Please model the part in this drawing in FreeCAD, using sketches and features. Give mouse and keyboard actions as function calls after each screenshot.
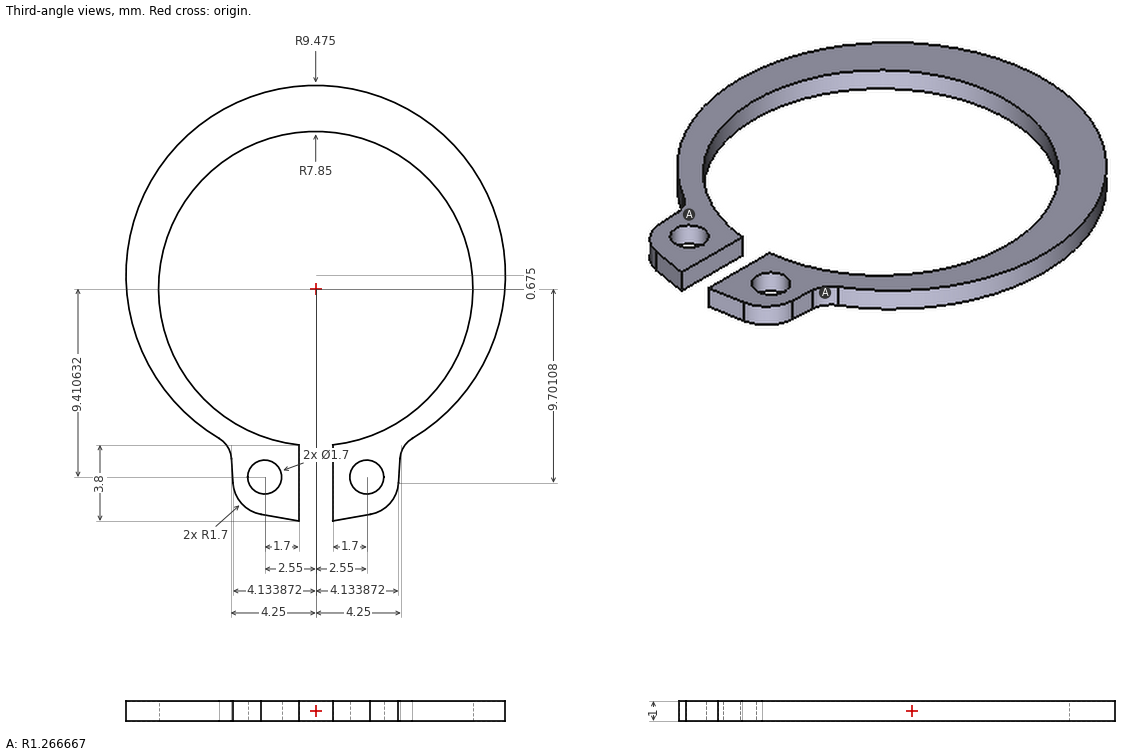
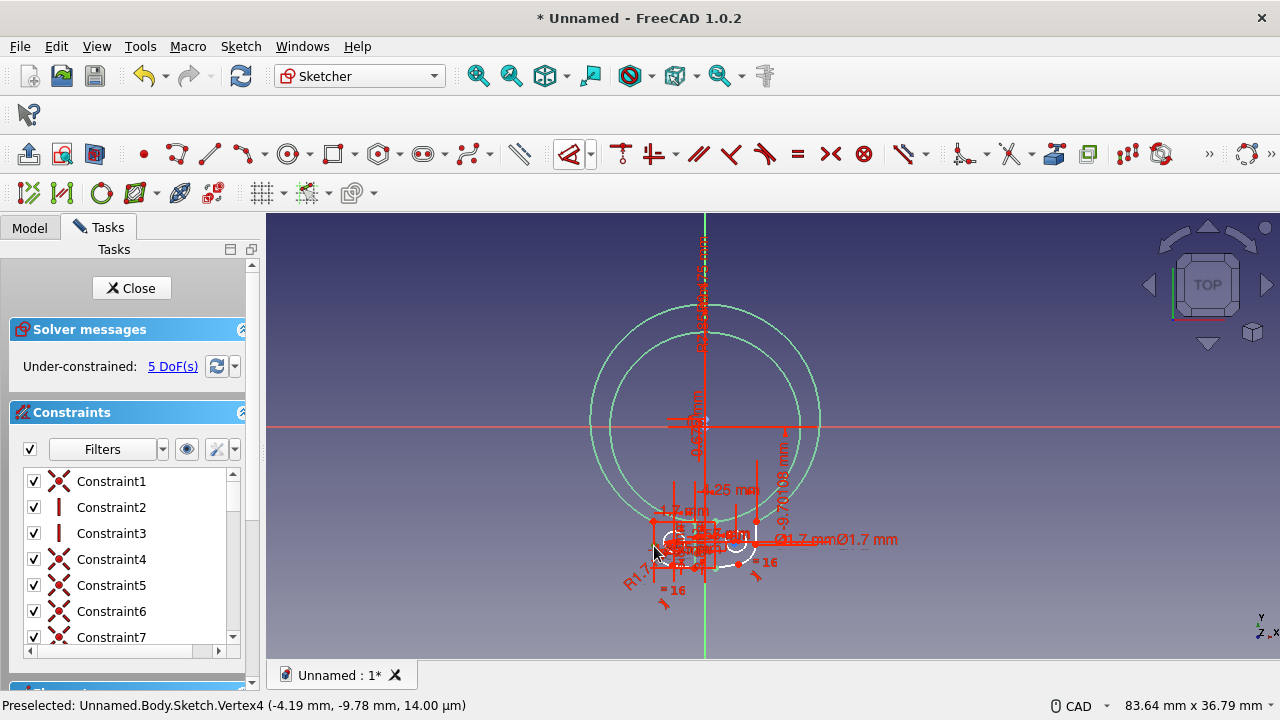
click(590, 154)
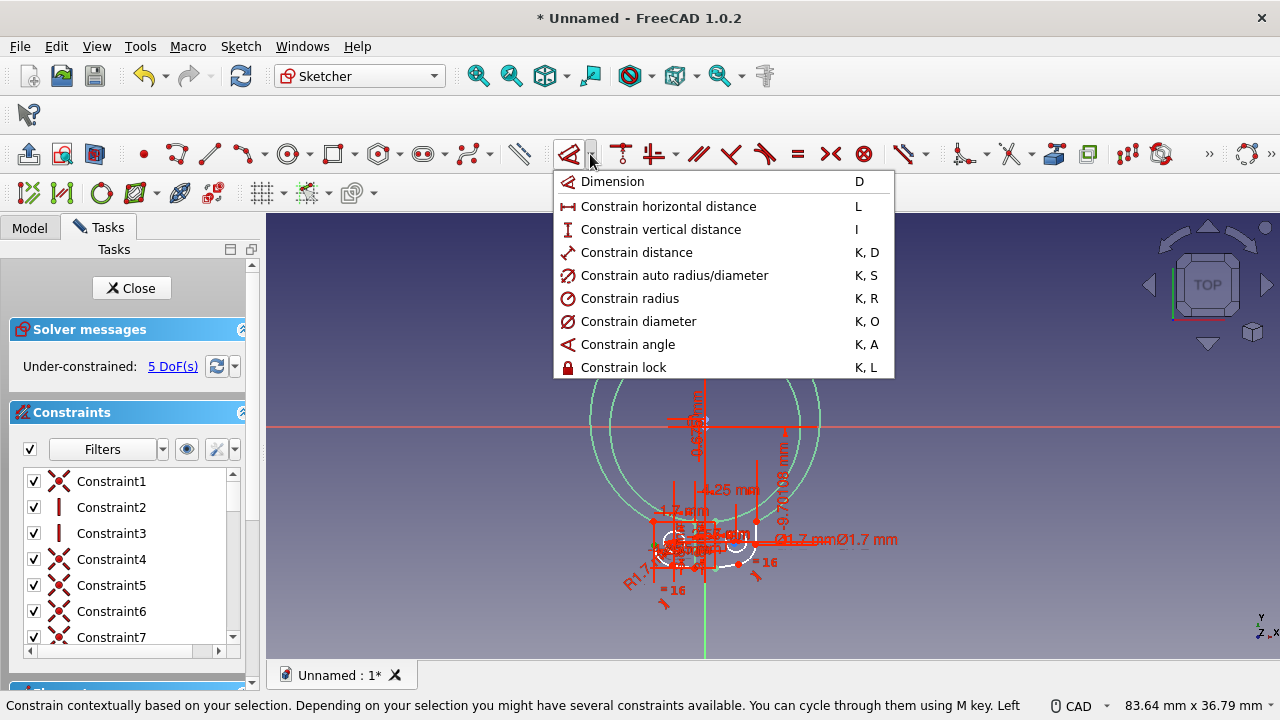
click(724, 230)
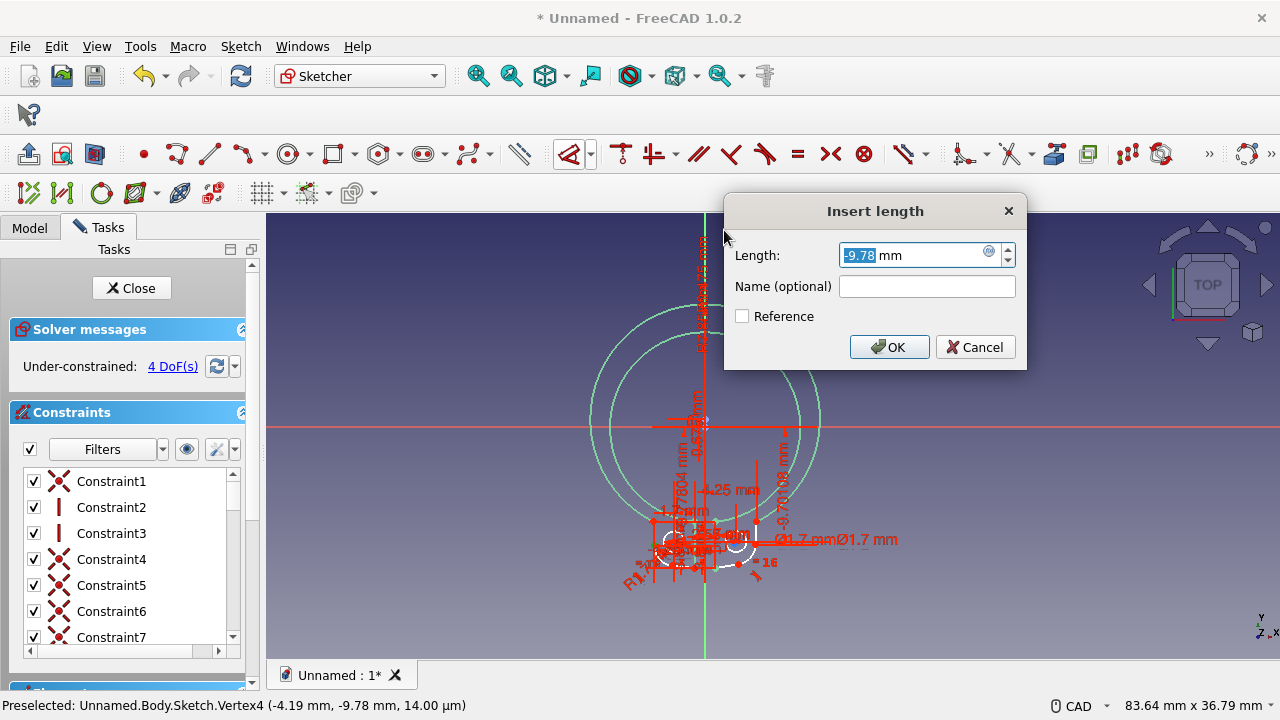
text(-9.70108)
key(Return)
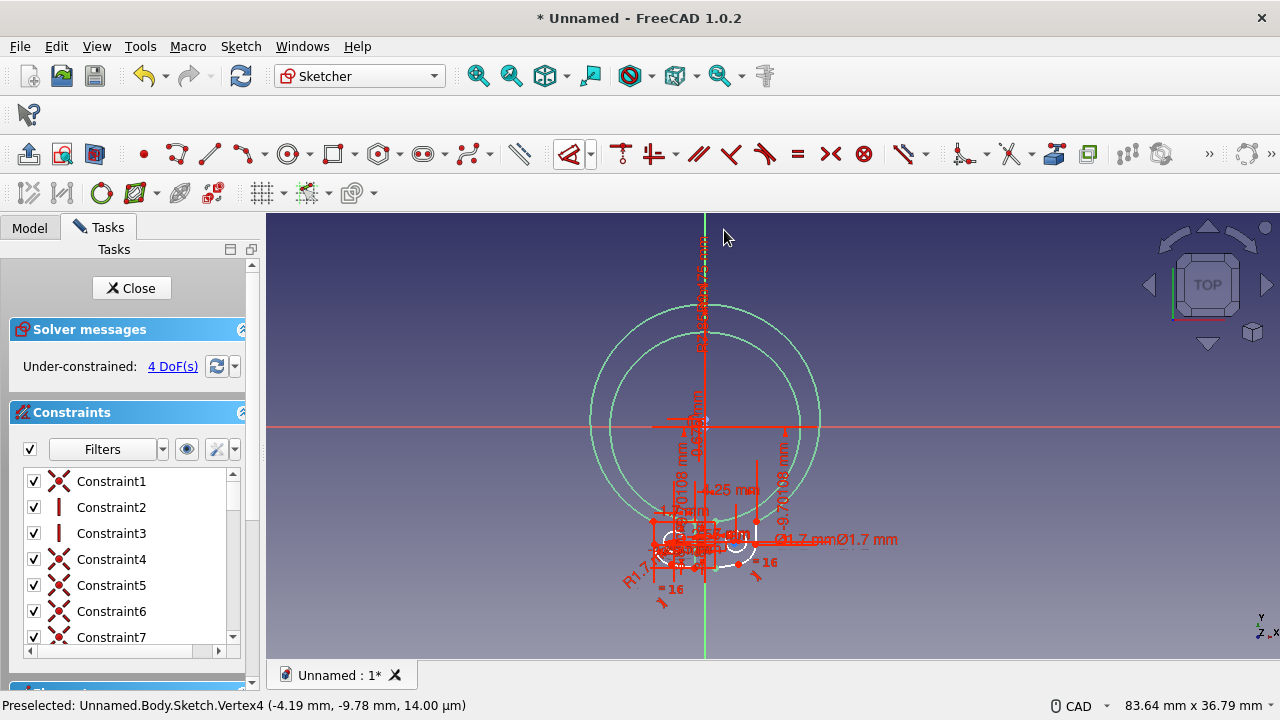
scroll(674, 542, up, 8)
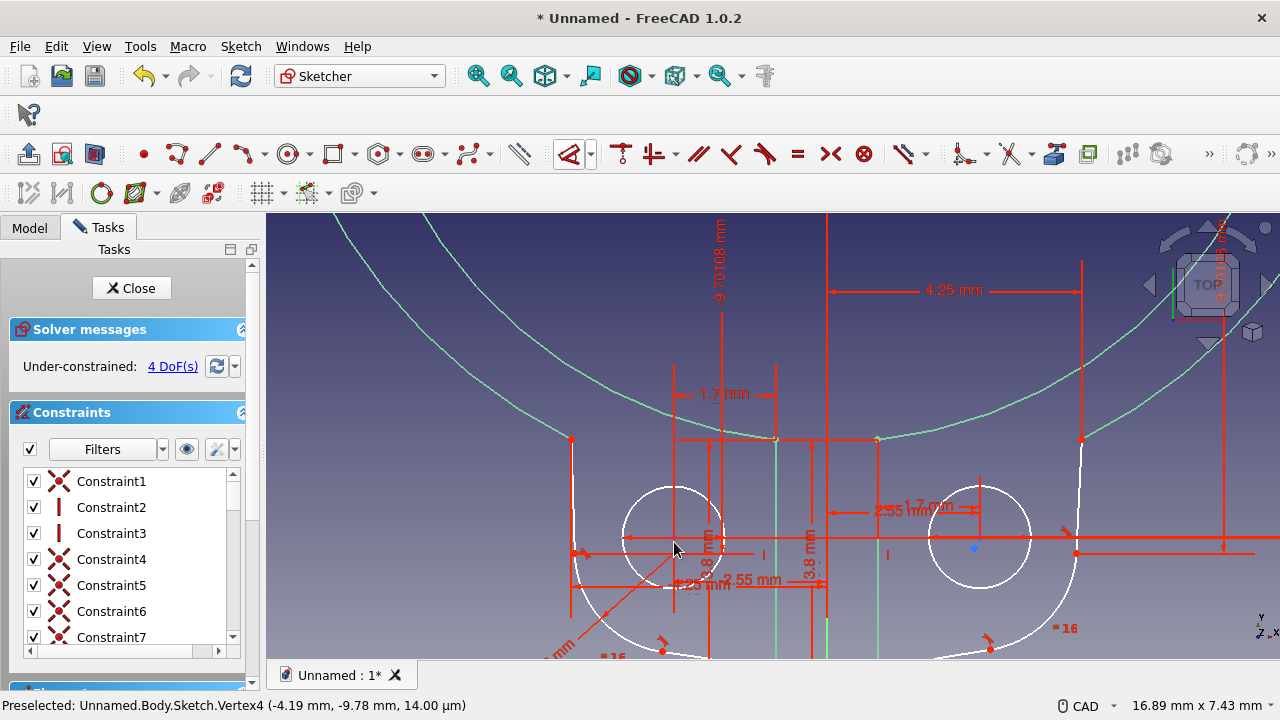
click(674, 538)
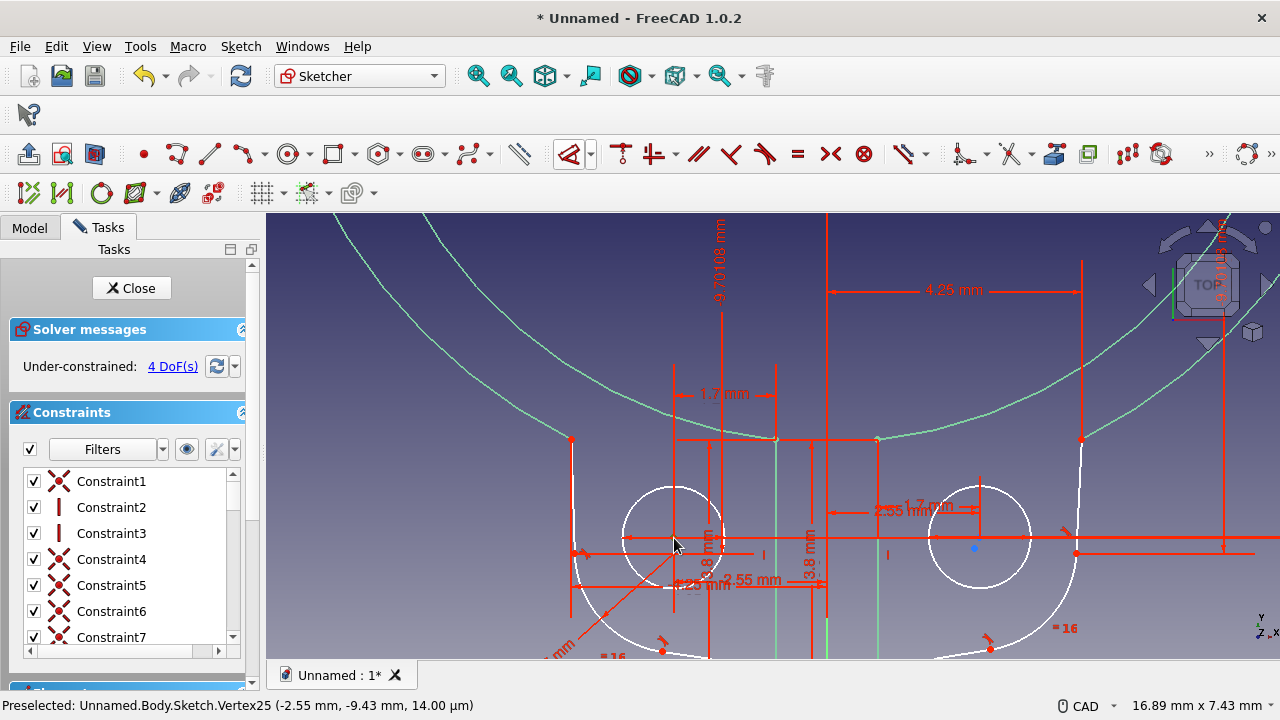
click(590, 154)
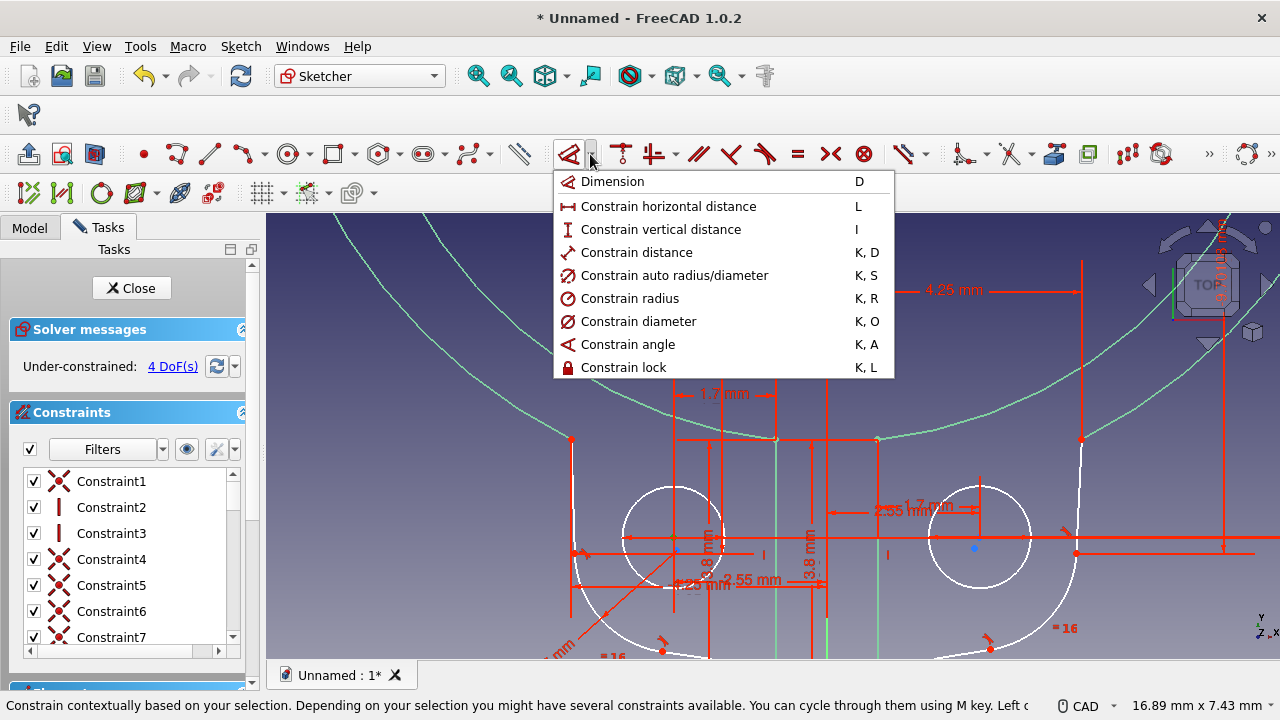
click(724, 230)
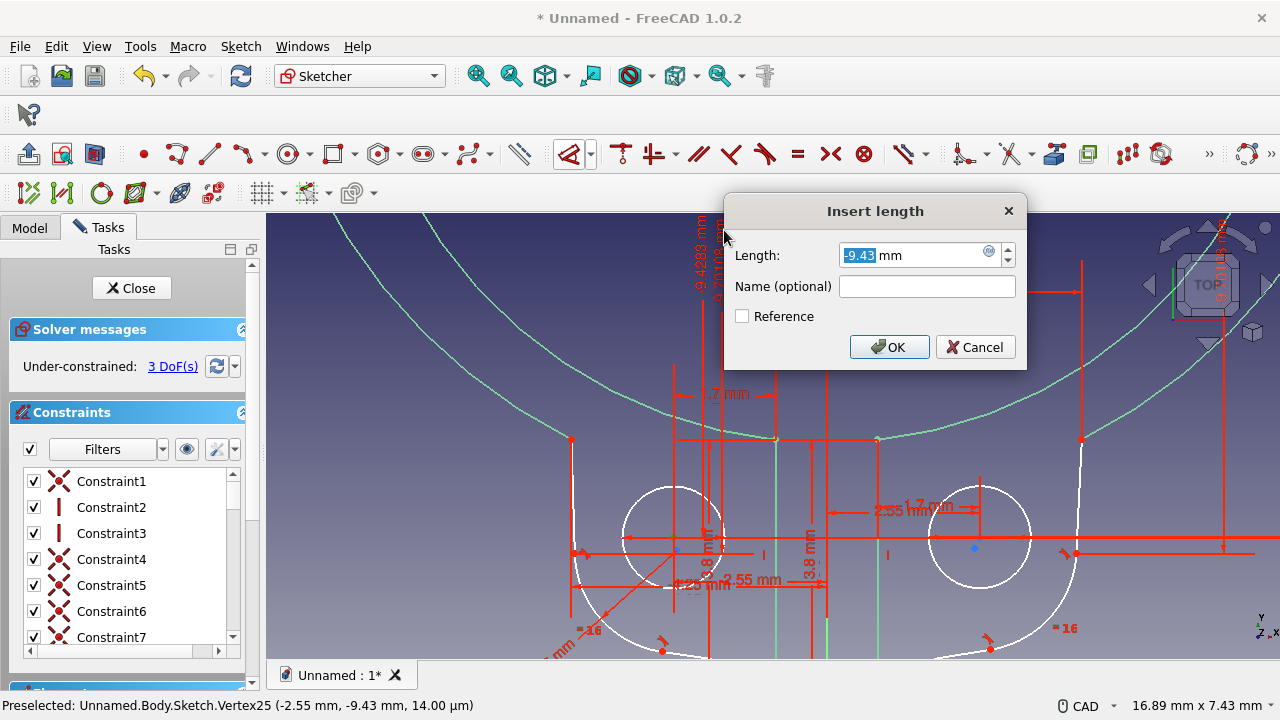
text(-9.410632)
key(Return)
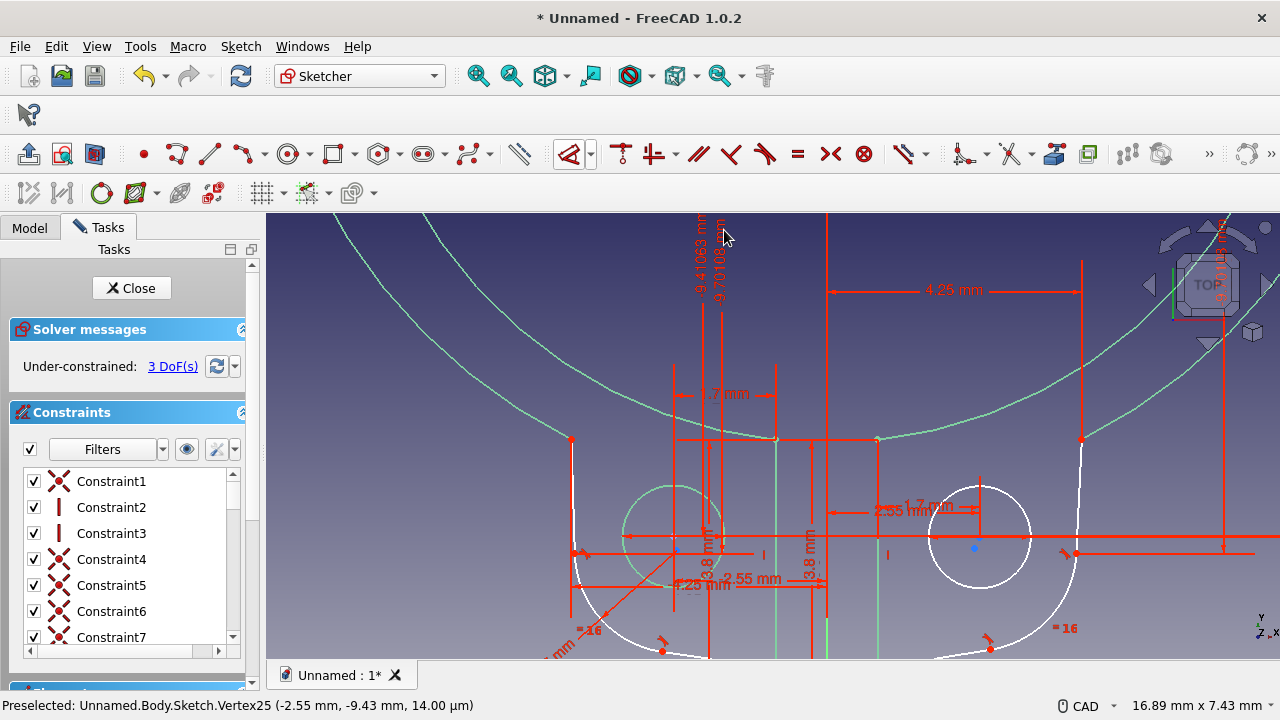
click(980, 537)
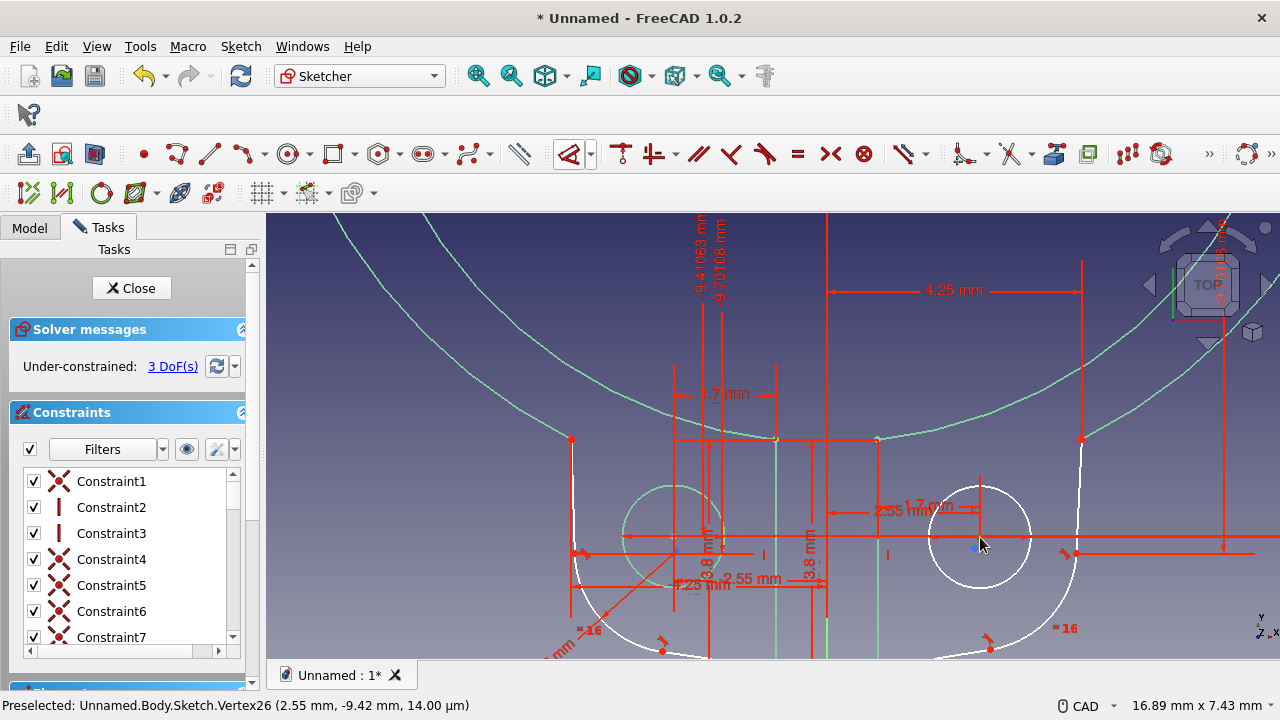
key(i)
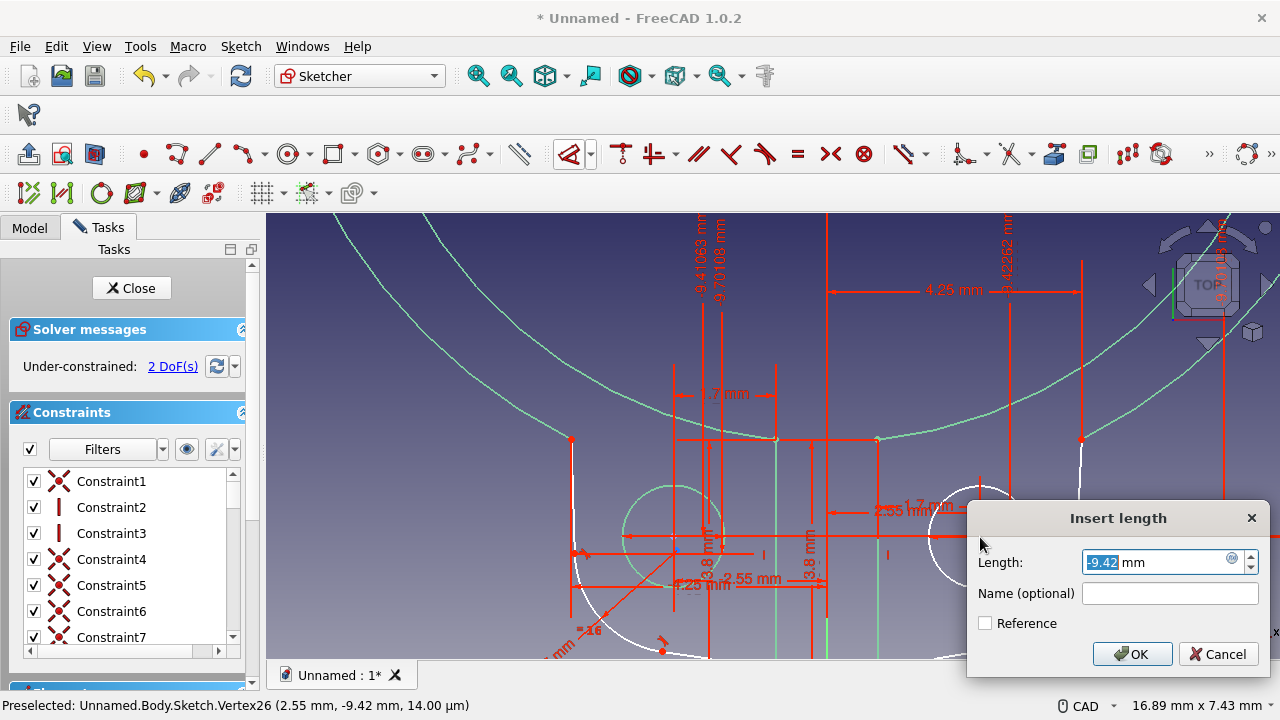
text(-9.410632)
key(Return)